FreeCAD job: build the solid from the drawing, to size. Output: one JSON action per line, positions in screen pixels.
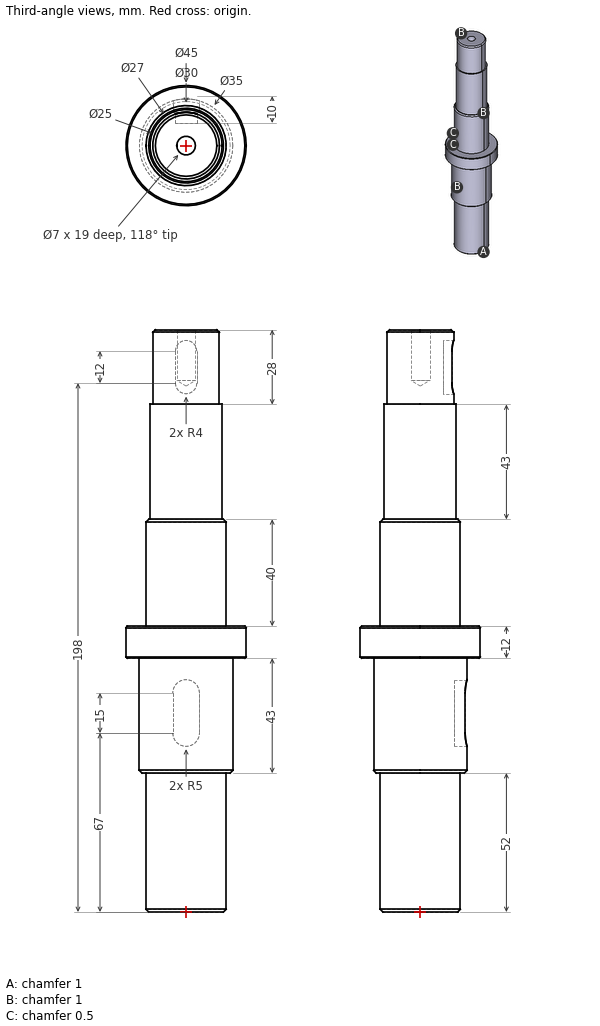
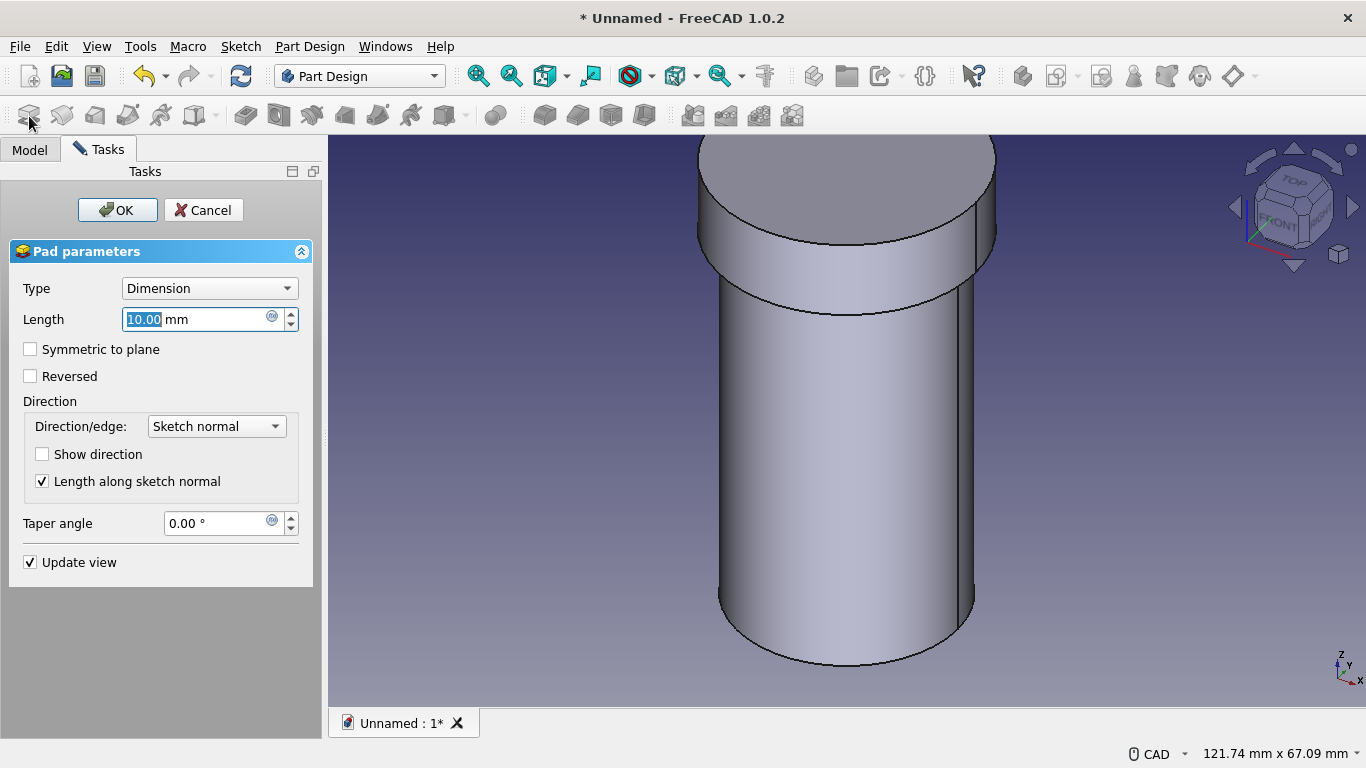
{"action": "type", "text": "43"}
{"action": "key", "text": "Tab"}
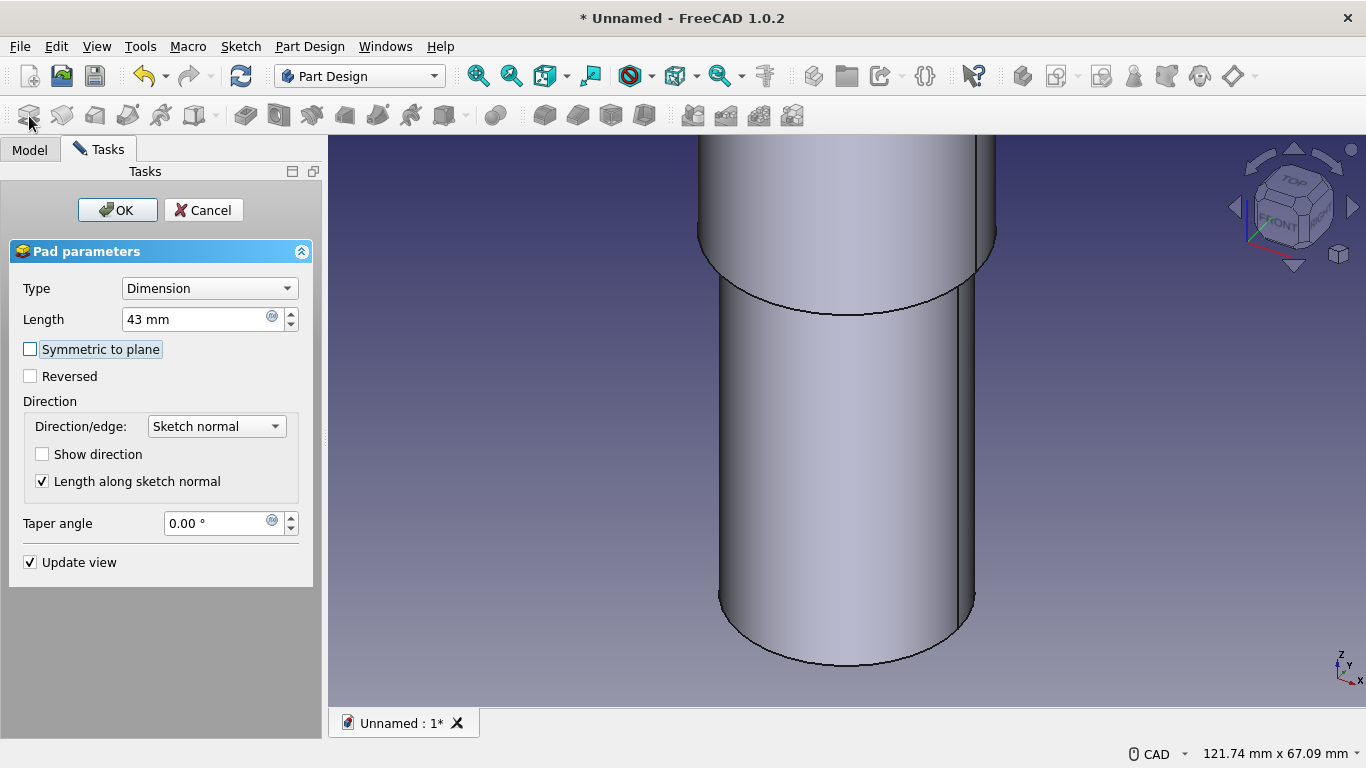
{"action": "left_click", "coordinate": [118, 210]}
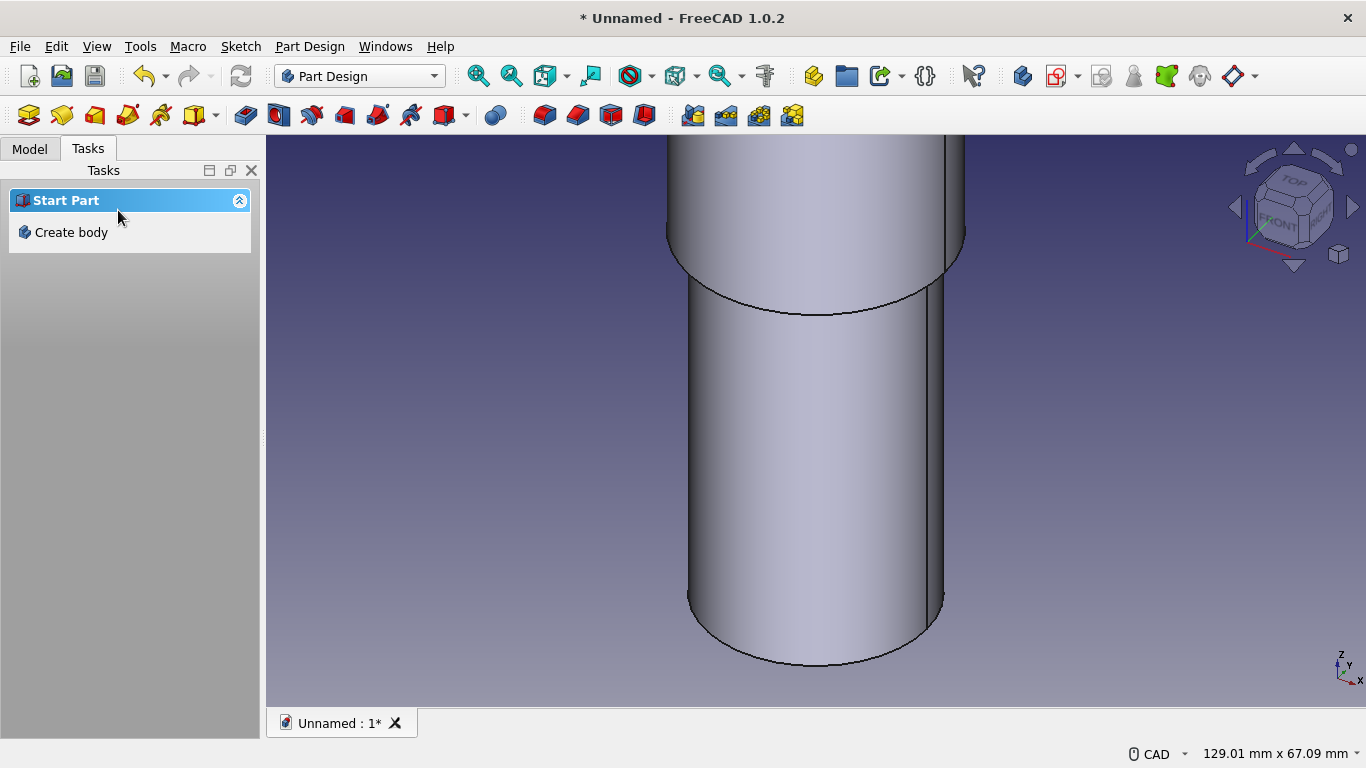
{"action": "key", "text": "v f"}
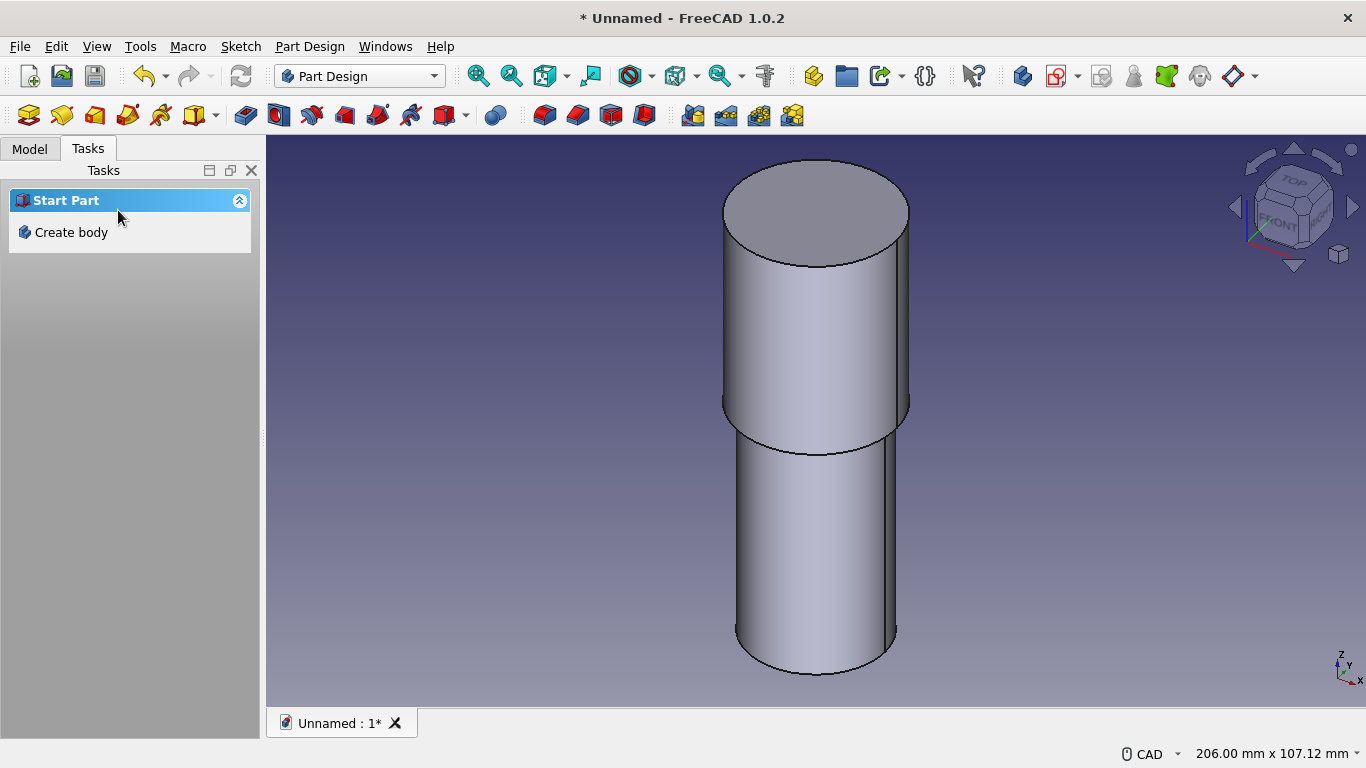
{"action": "left_click", "coordinate": [816, 212]}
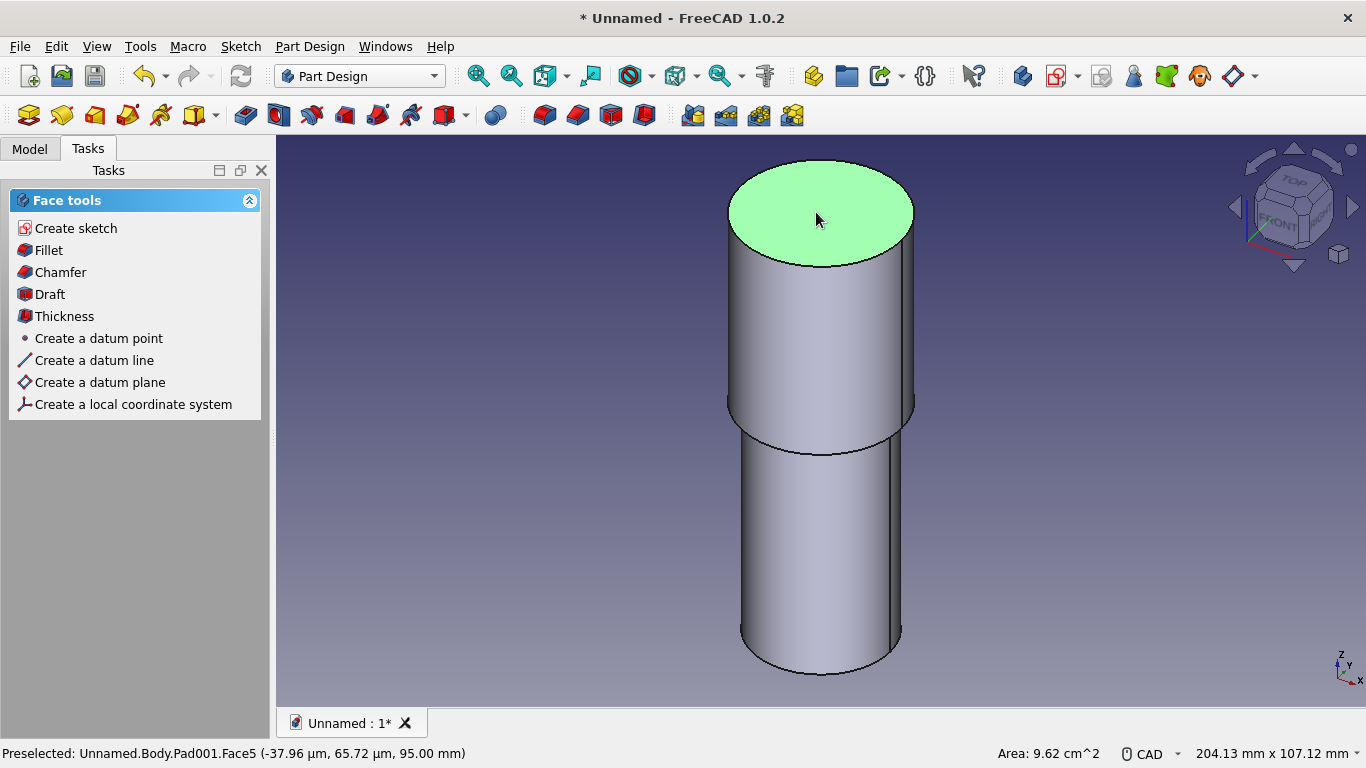
{"action": "left_click", "coordinate": [1056, 76]}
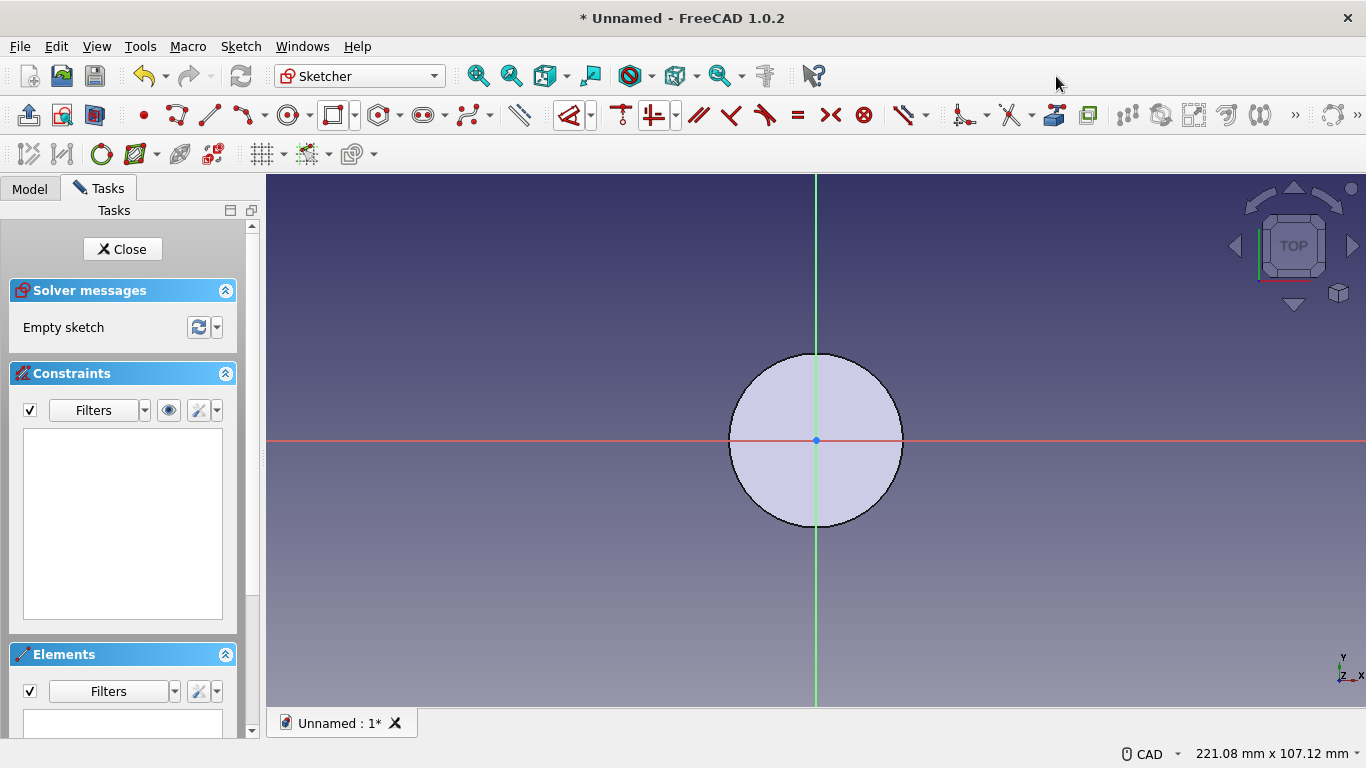
{"action": "scroll", "coordinate": [955, 440], "scroll_direction": "up", "scroll_amount": 2}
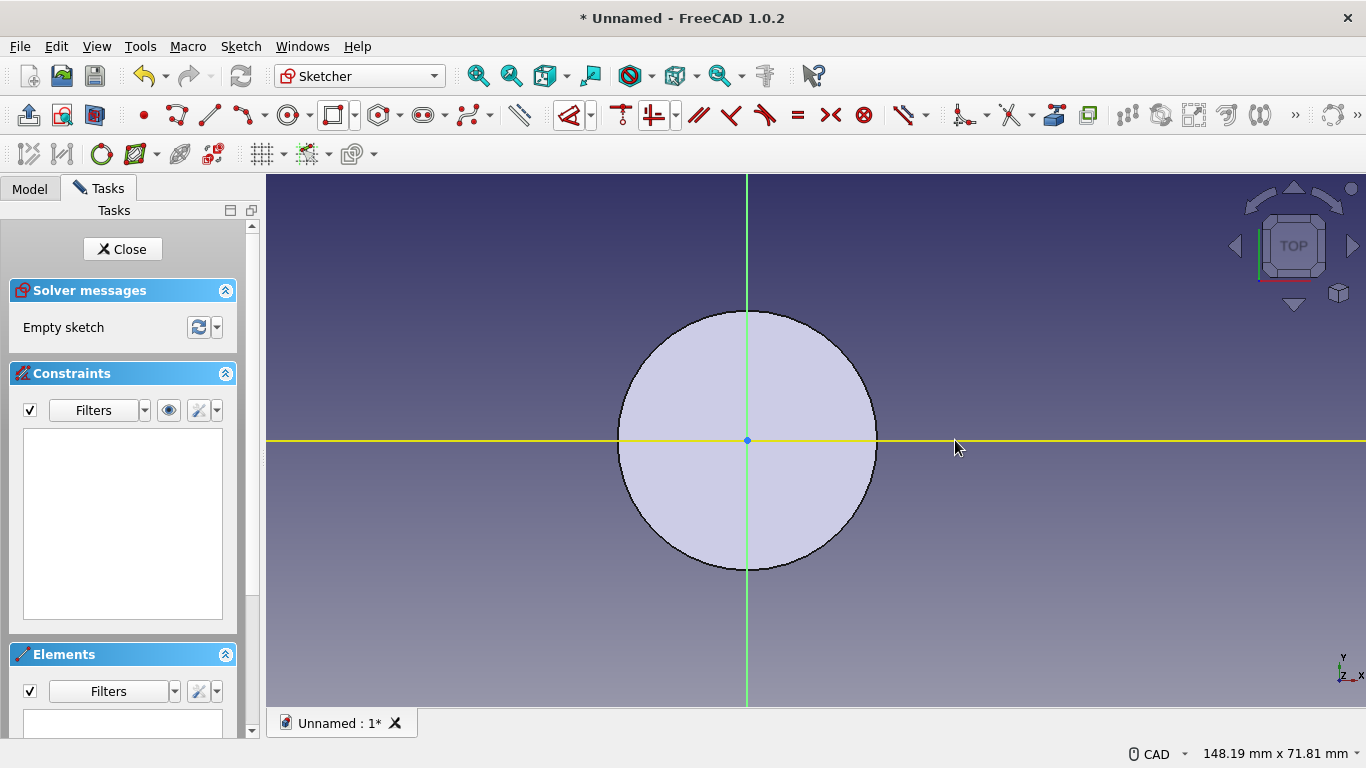
{"action": "key", "text": "g c"}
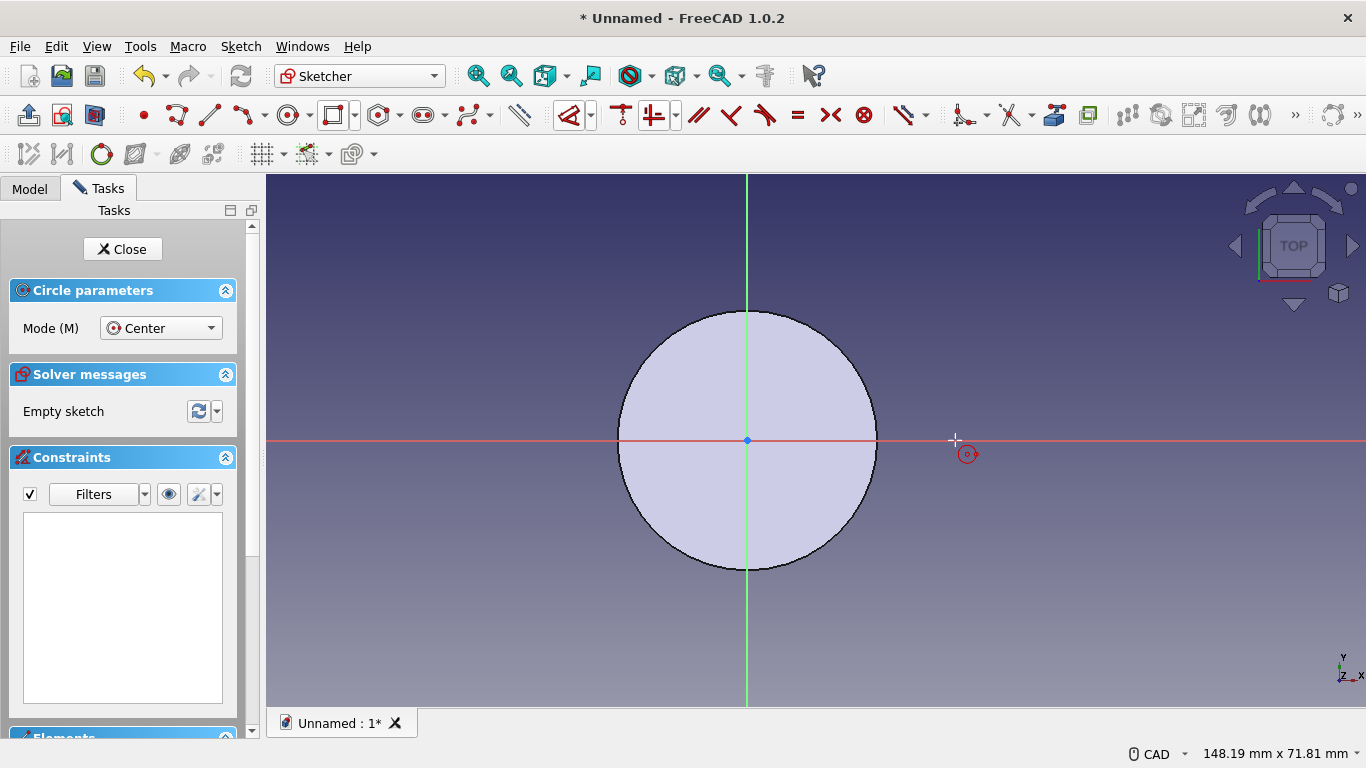
{"action": "left_click", "coordinate": [747, 440]}
{"action": "mouse_move", "coordinate": [865, 322]}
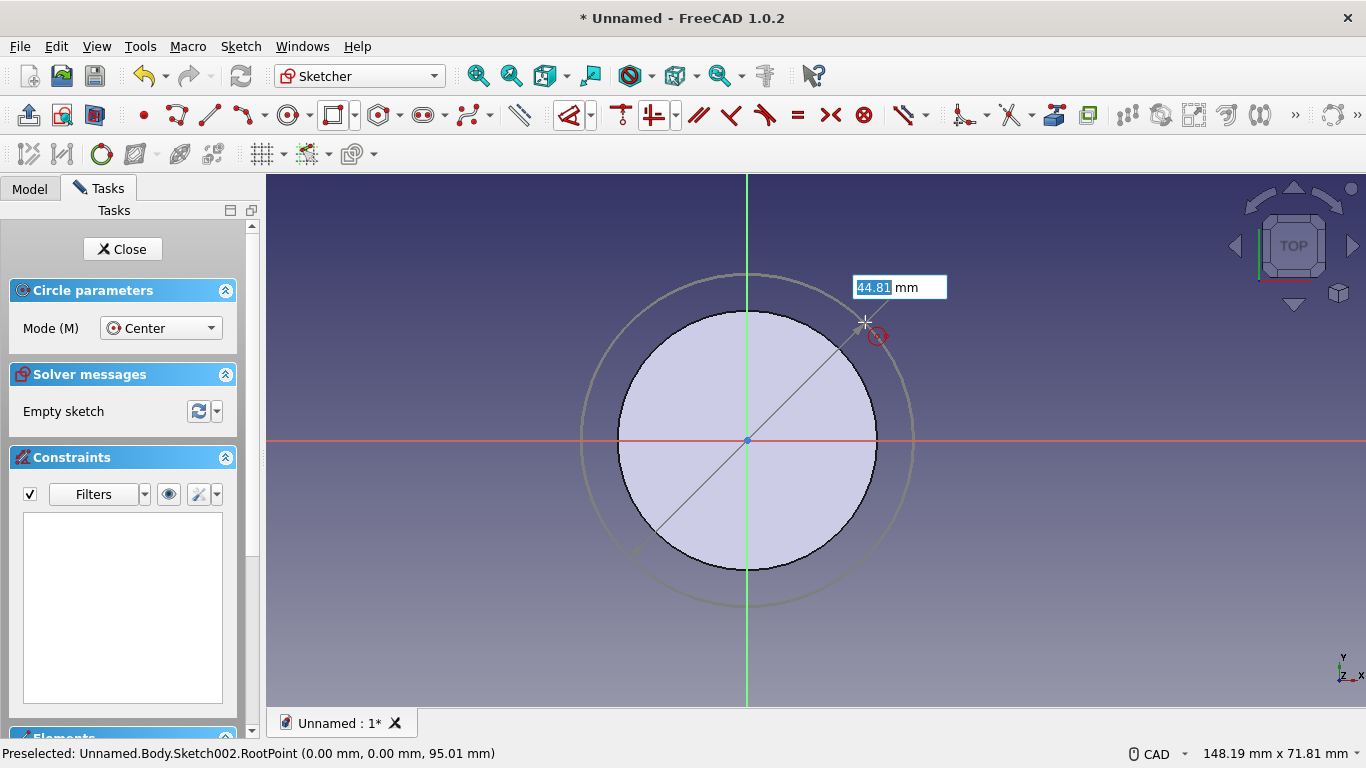
{"action": "type", "text": "45"}
{"action": "key", "text": "Return"}
{"action": "key", "text": "Escape"}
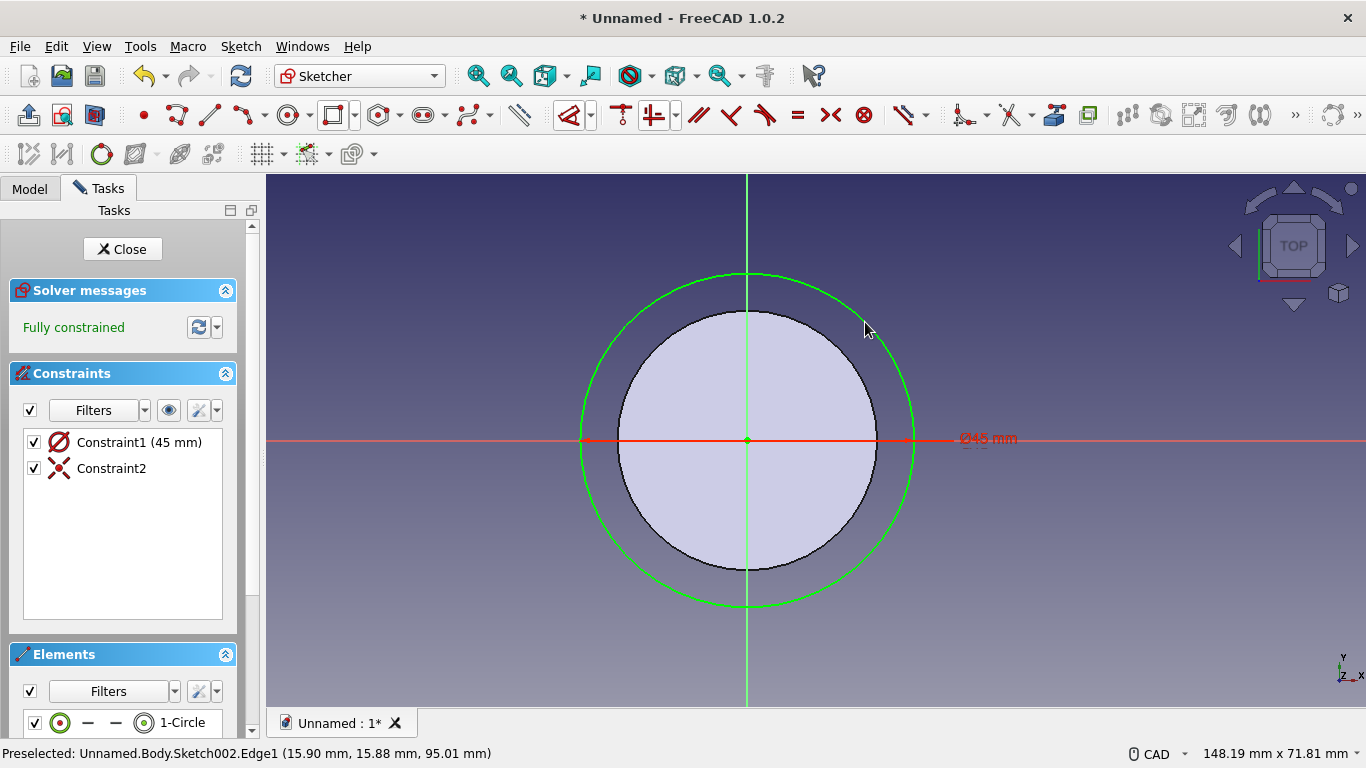
{"action": "left_click", "coordinate": [123, 249]}